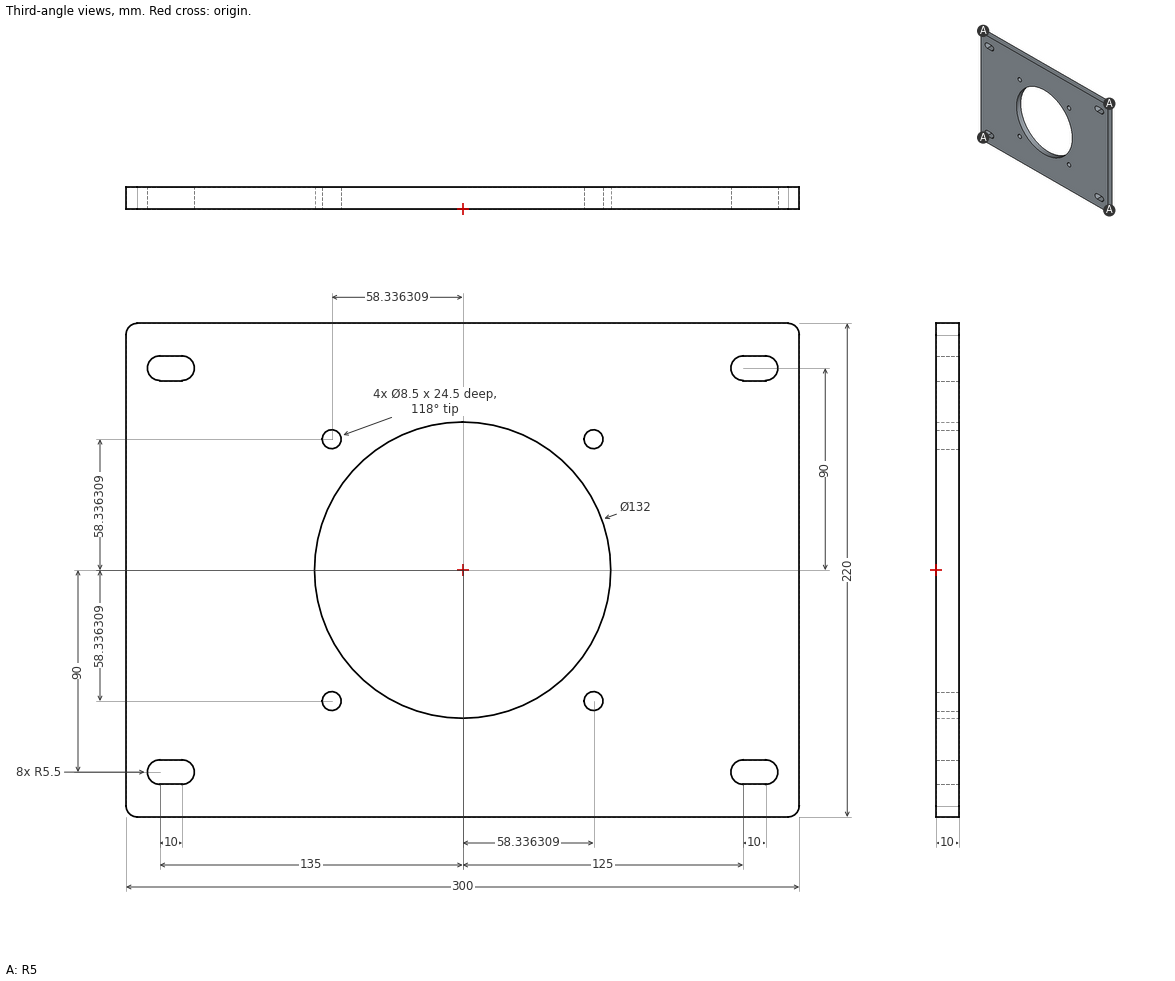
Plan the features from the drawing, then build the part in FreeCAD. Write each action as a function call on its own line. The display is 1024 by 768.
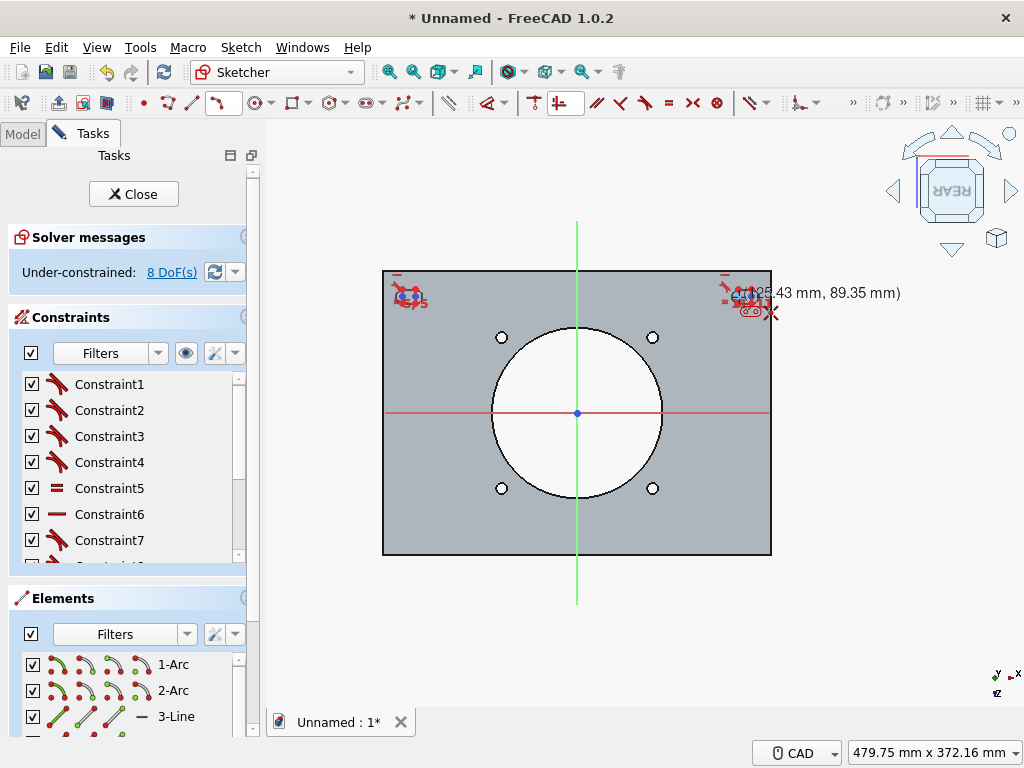
scroll(739, 530, up, 6)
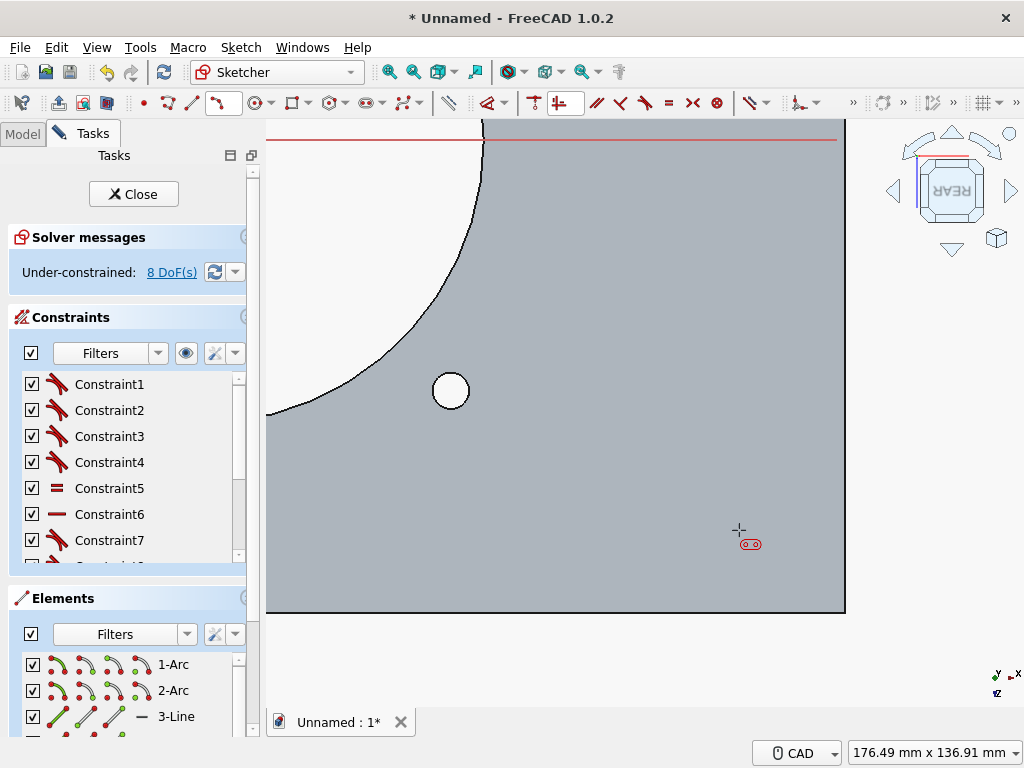
click(737, 527)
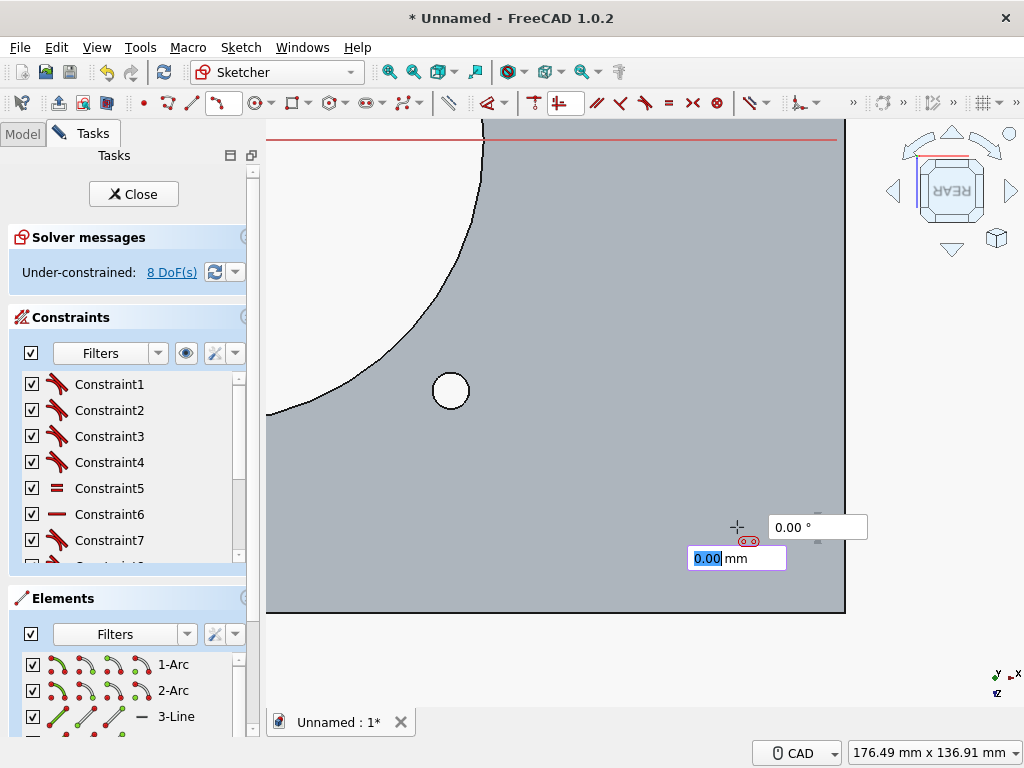
click(780, 527)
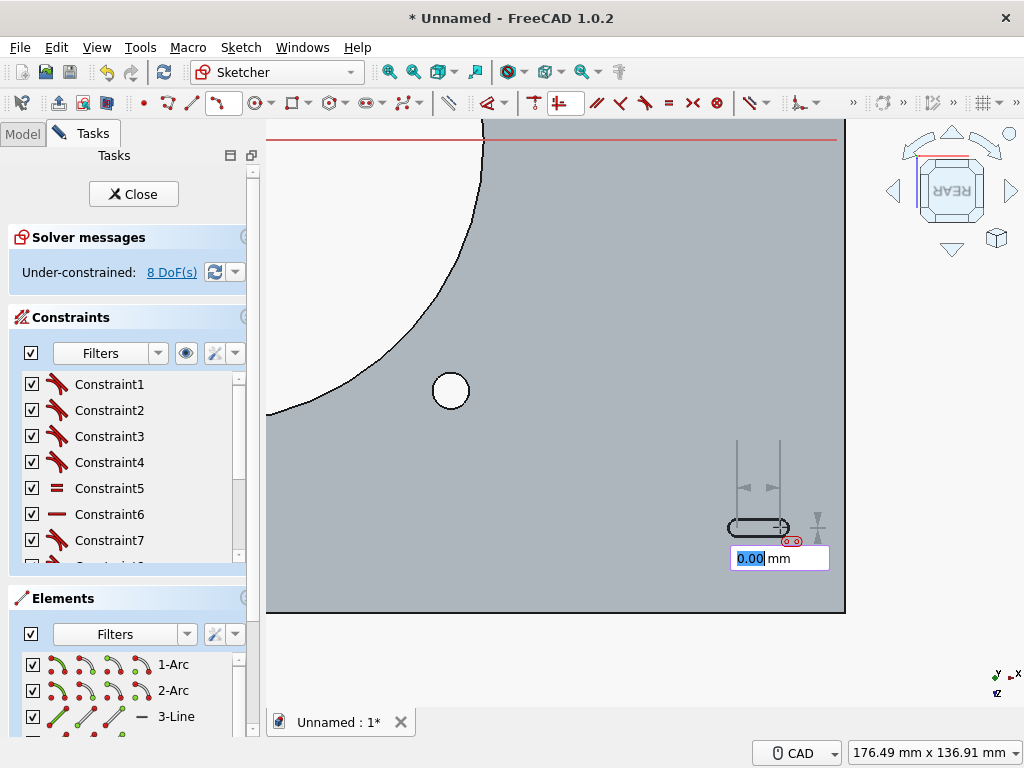
click(759, 550)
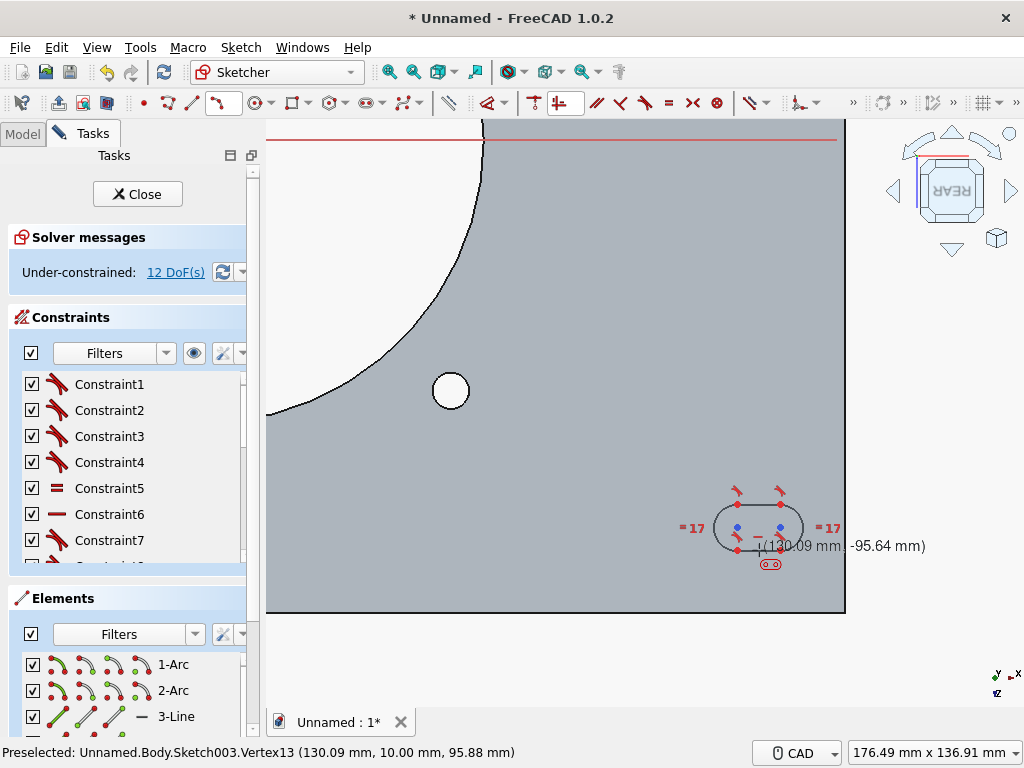
scroll(739, 531, down, 6)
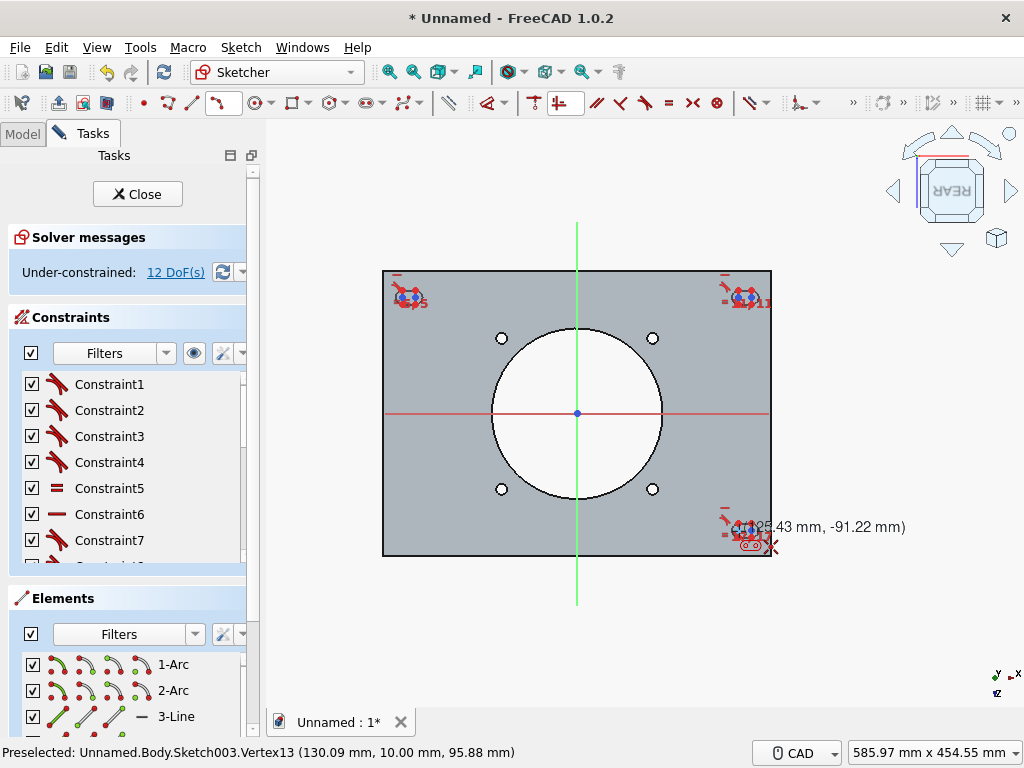
scroll(403, 530, up, 6)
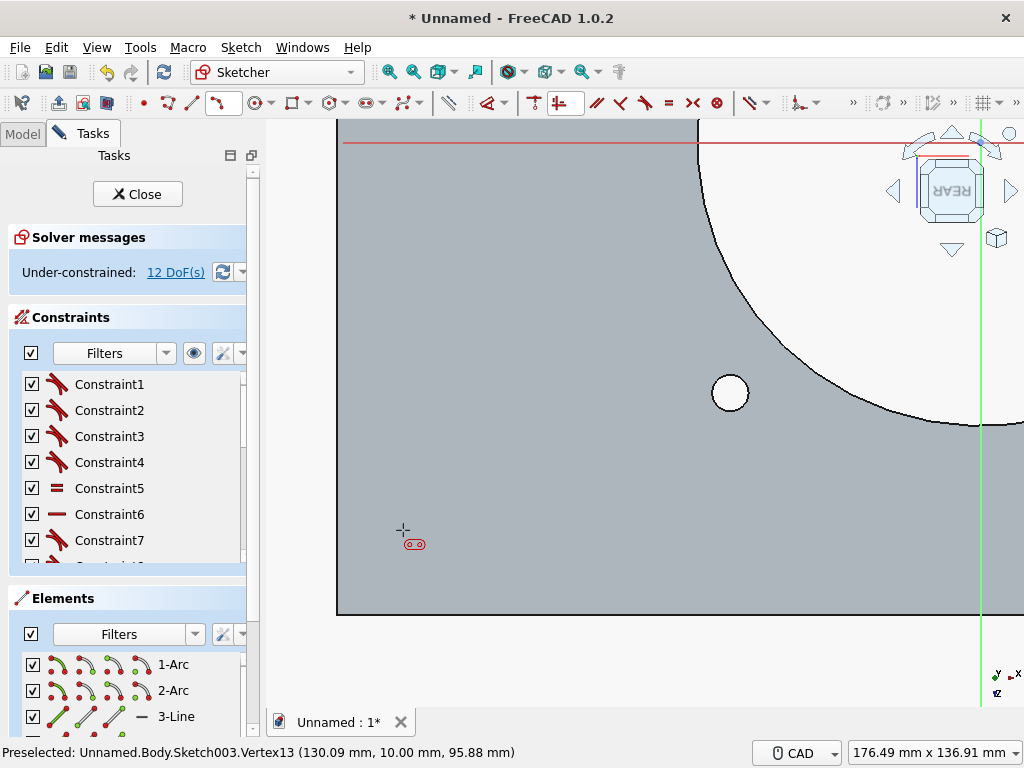
click(401, 529)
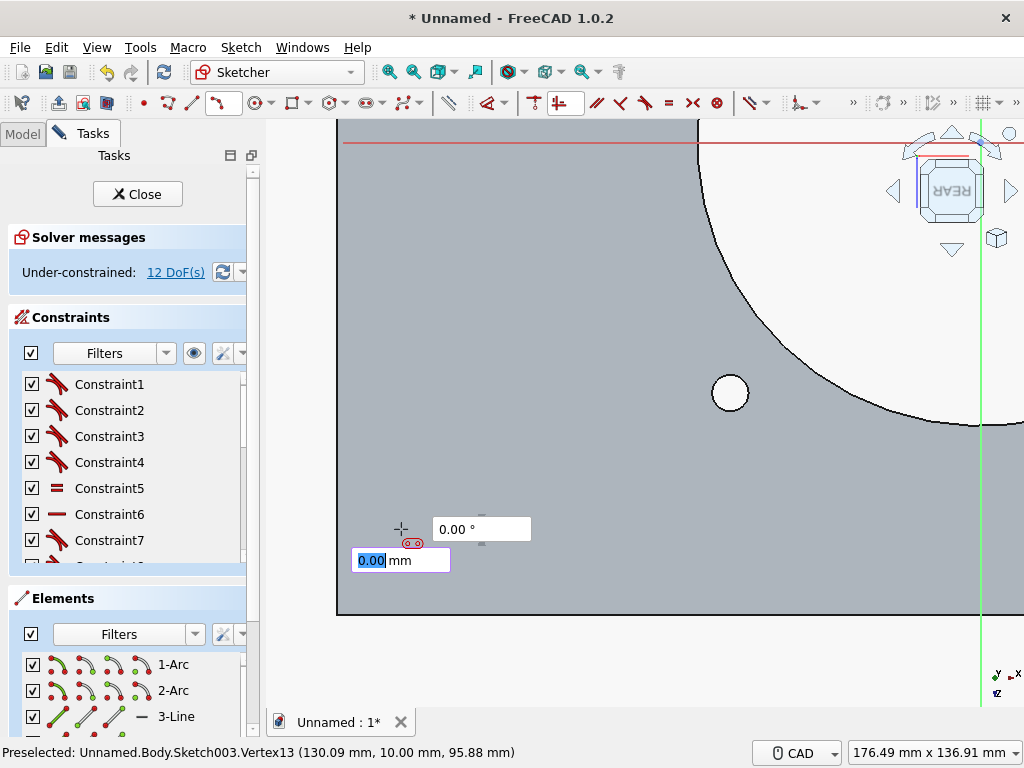
click(444, 529)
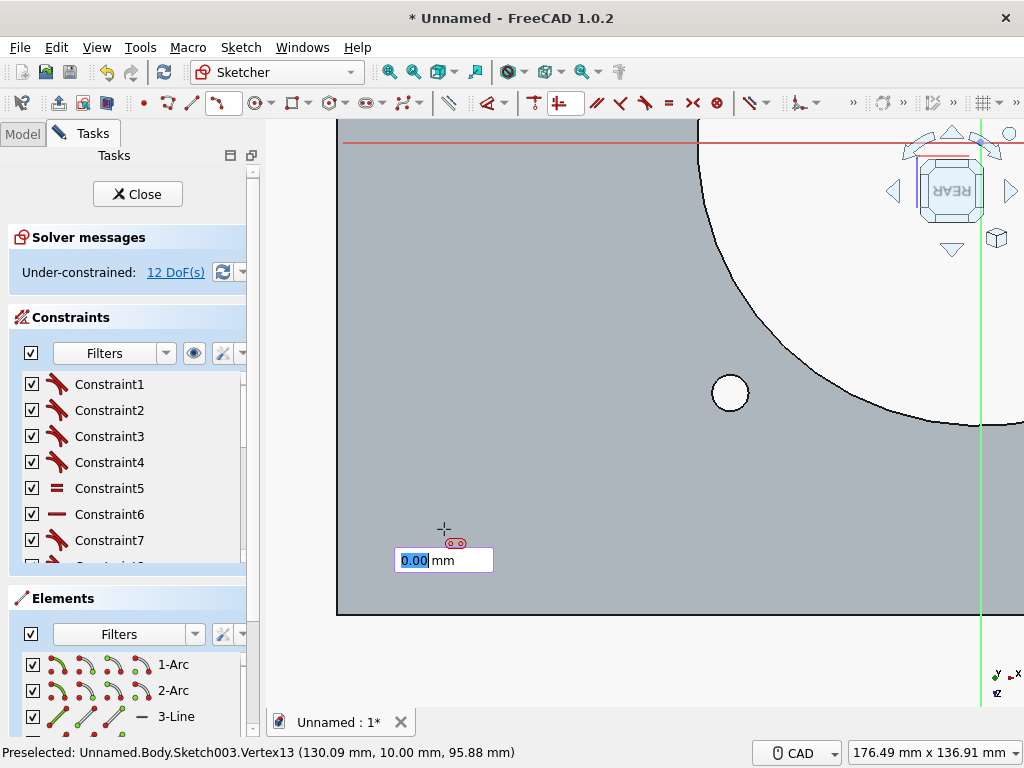
click(423, 553)
key(Escape)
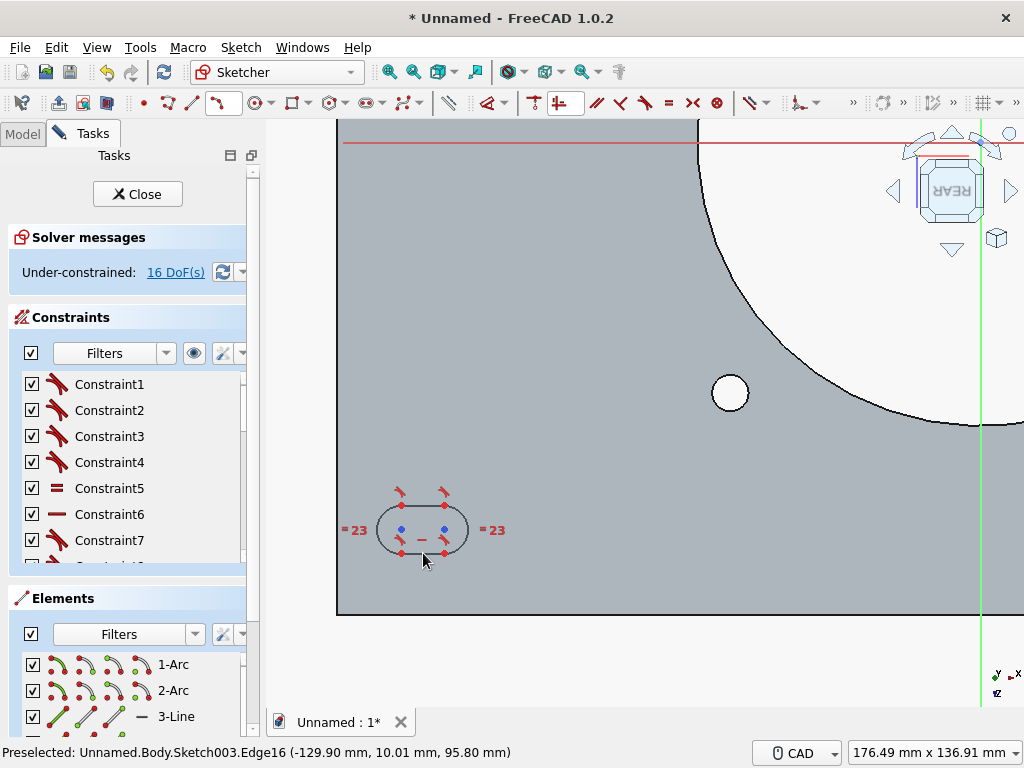
scroll(402, 530, down, 6)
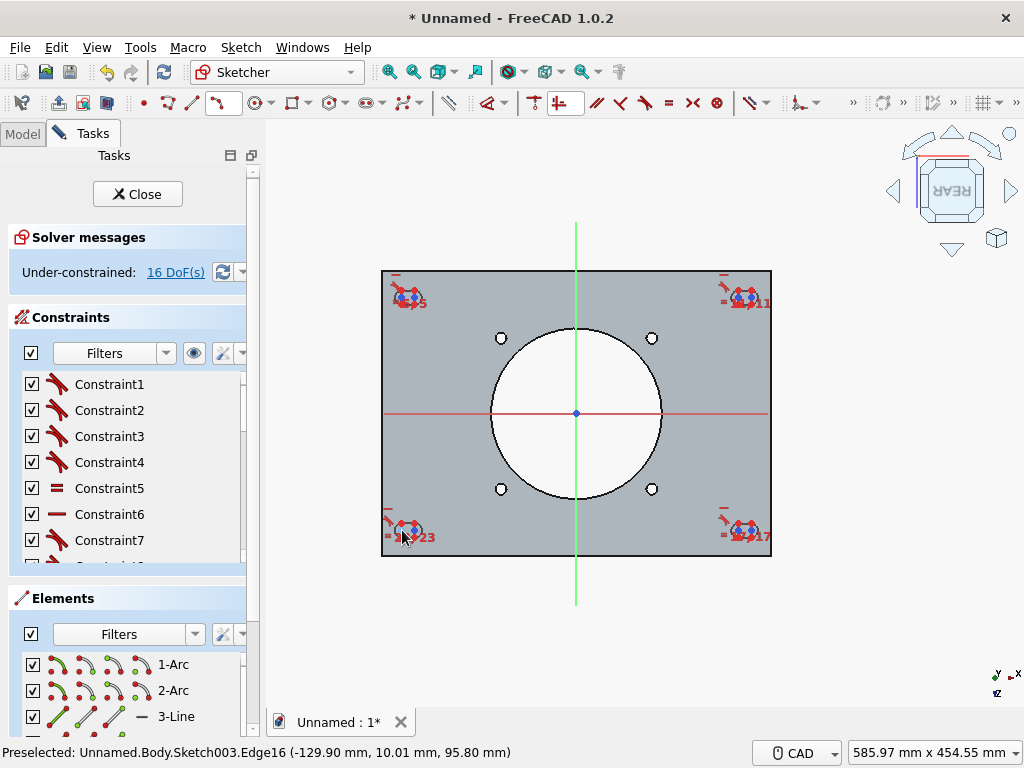
scroll(396, 294, up, 4)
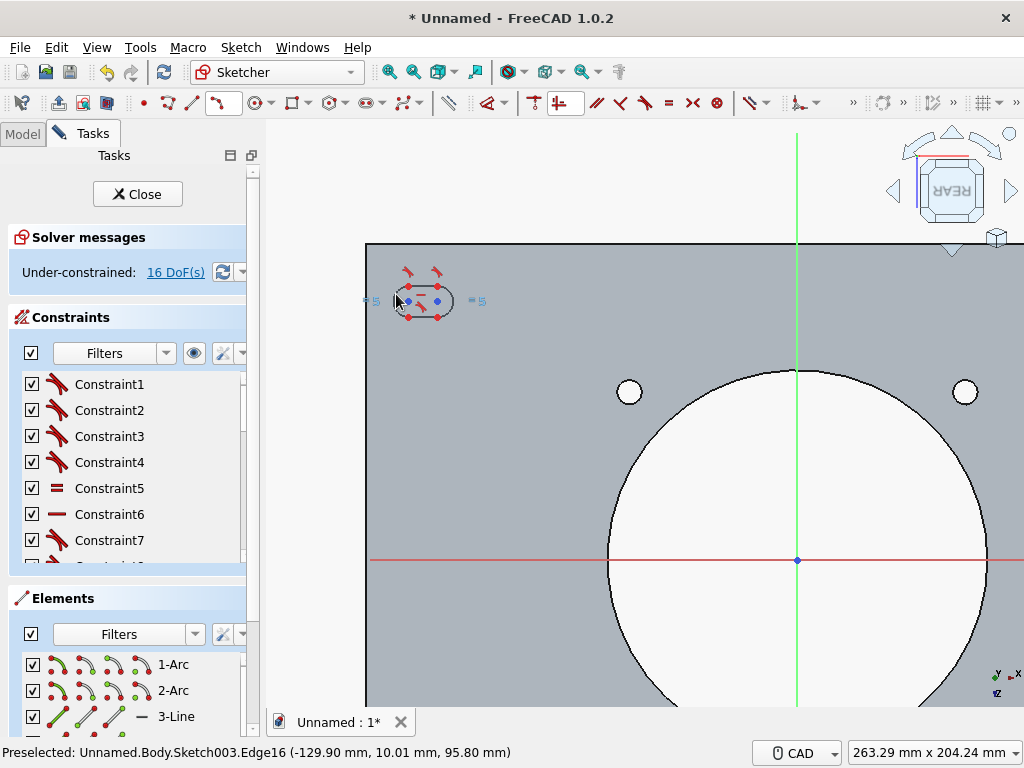
click(397, 293)